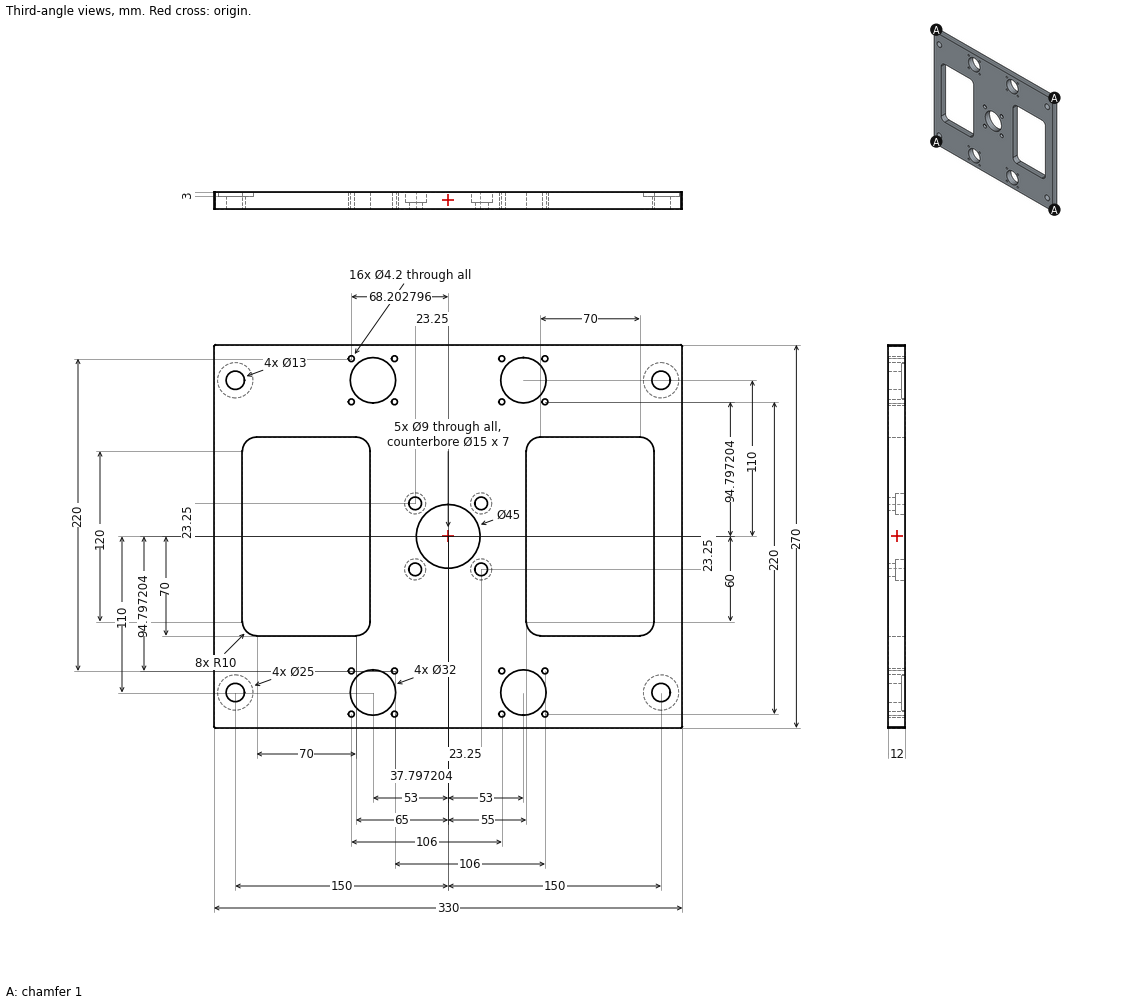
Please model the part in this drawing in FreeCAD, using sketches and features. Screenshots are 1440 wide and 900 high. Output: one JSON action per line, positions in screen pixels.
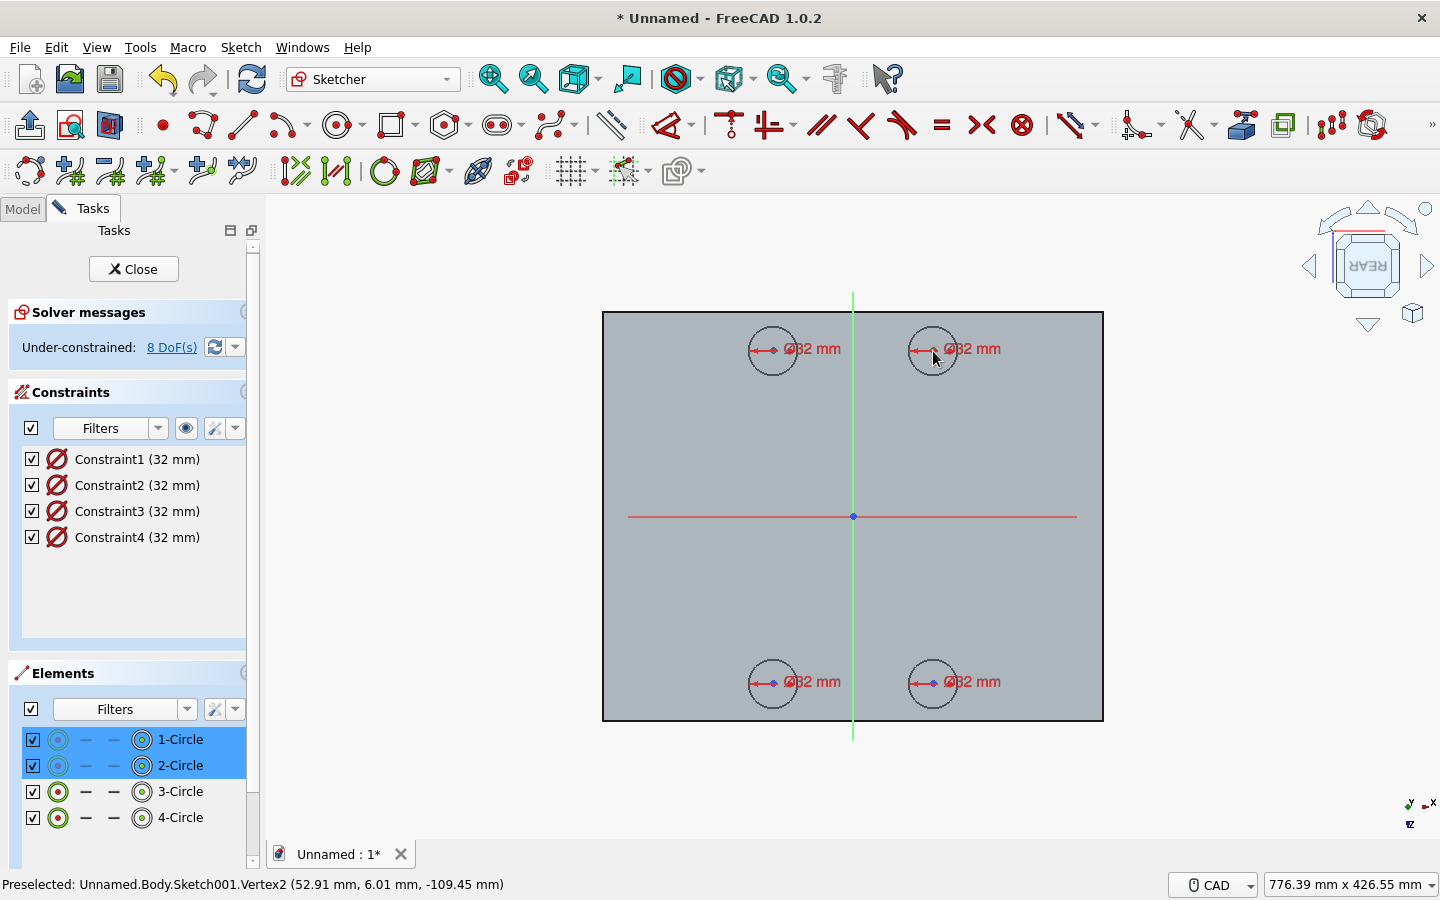
{"action": "left_click", "coordinate": [796, 126]}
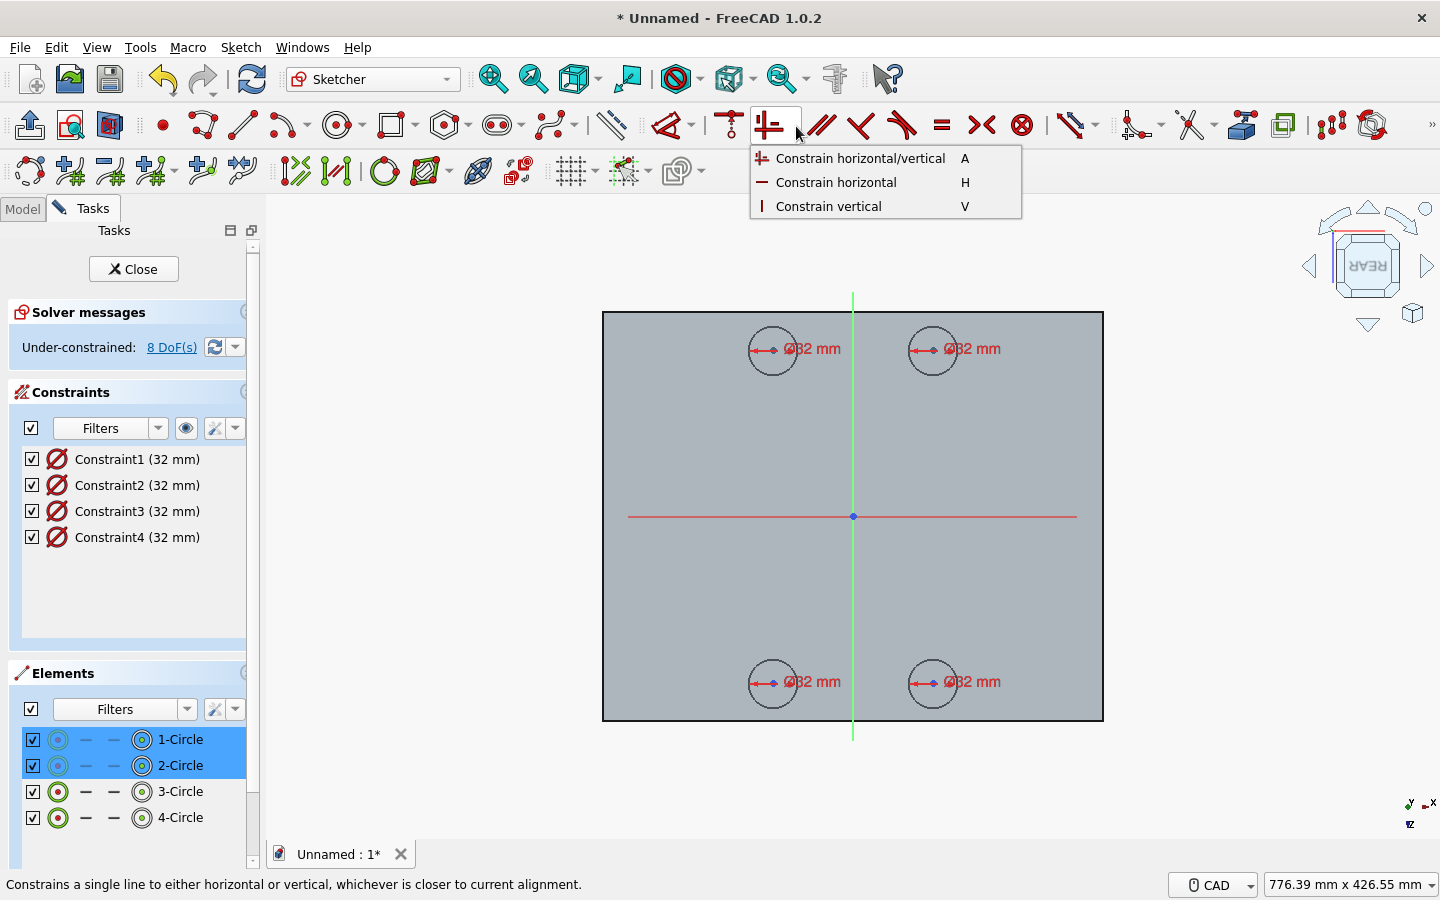
{"action": "left_click", "coordinate": [886, 182]}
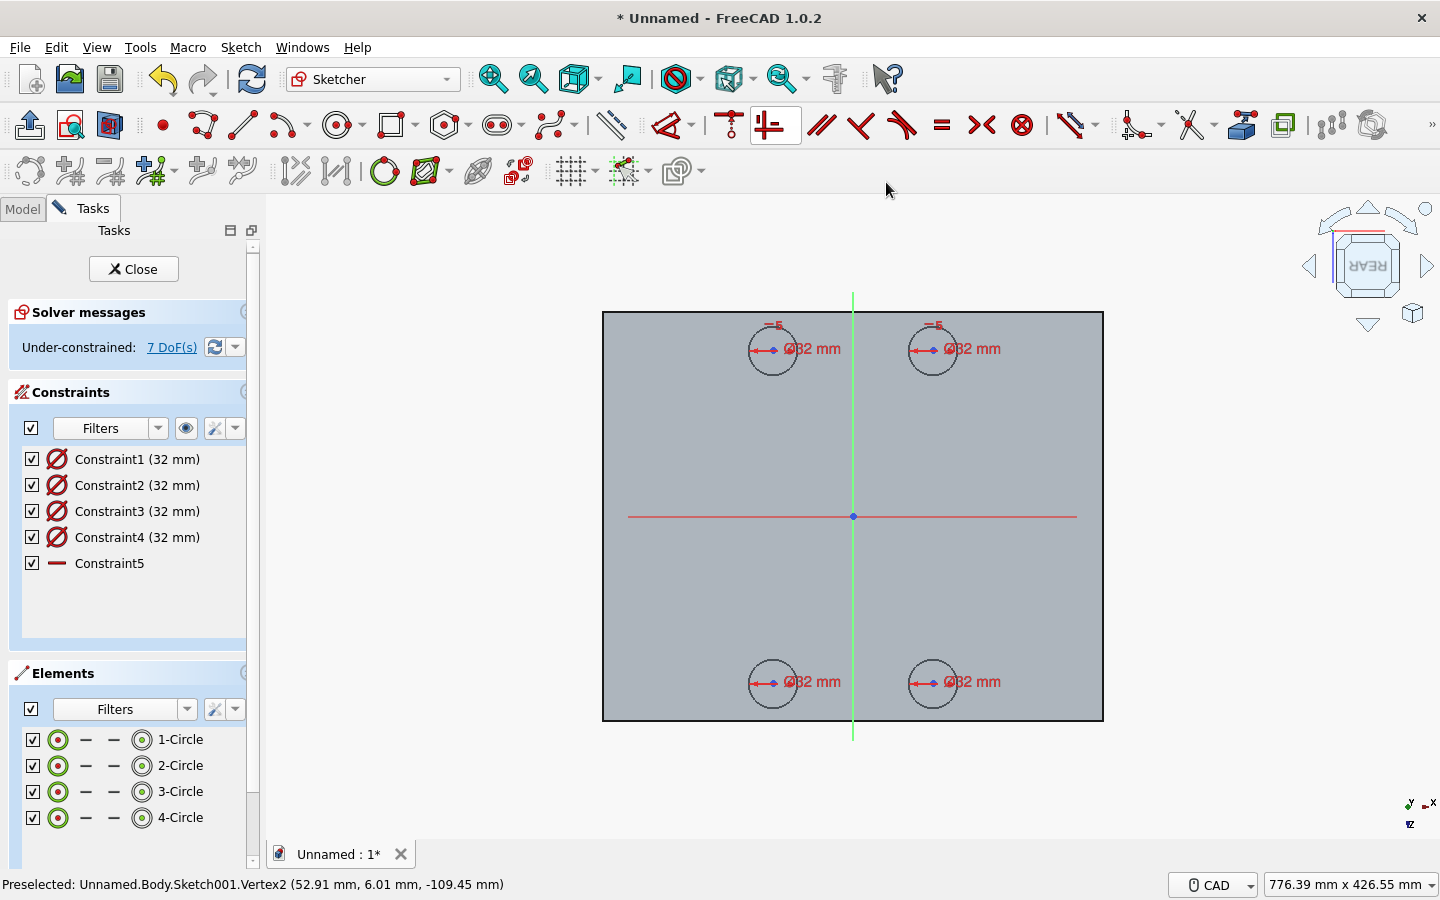
{"action": "left_click", "coordinate": [933, 351]}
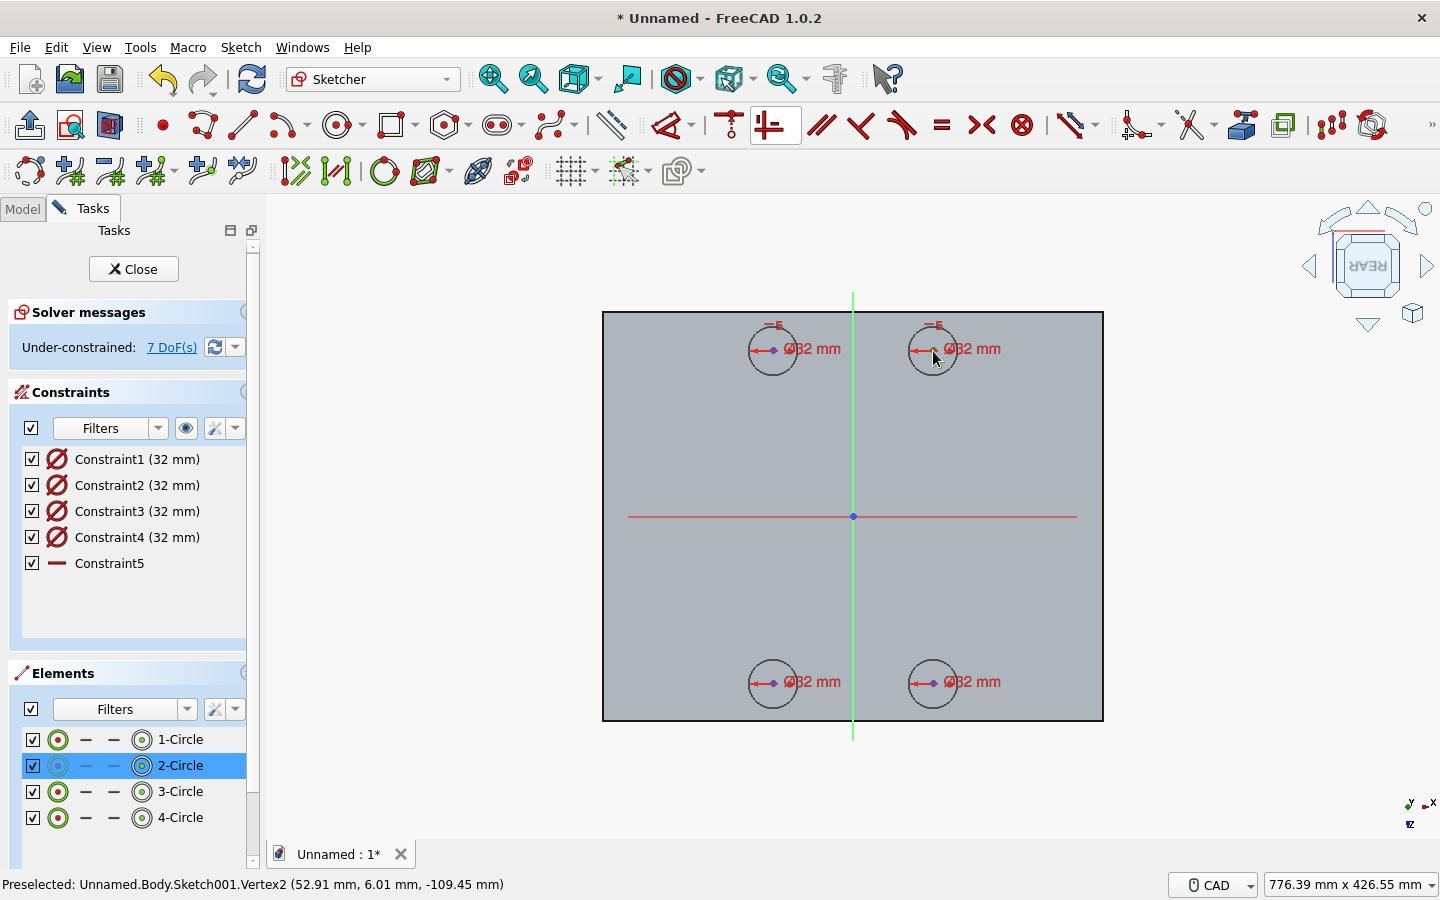
{"action": "left_click", "coordinate": [933, 684]}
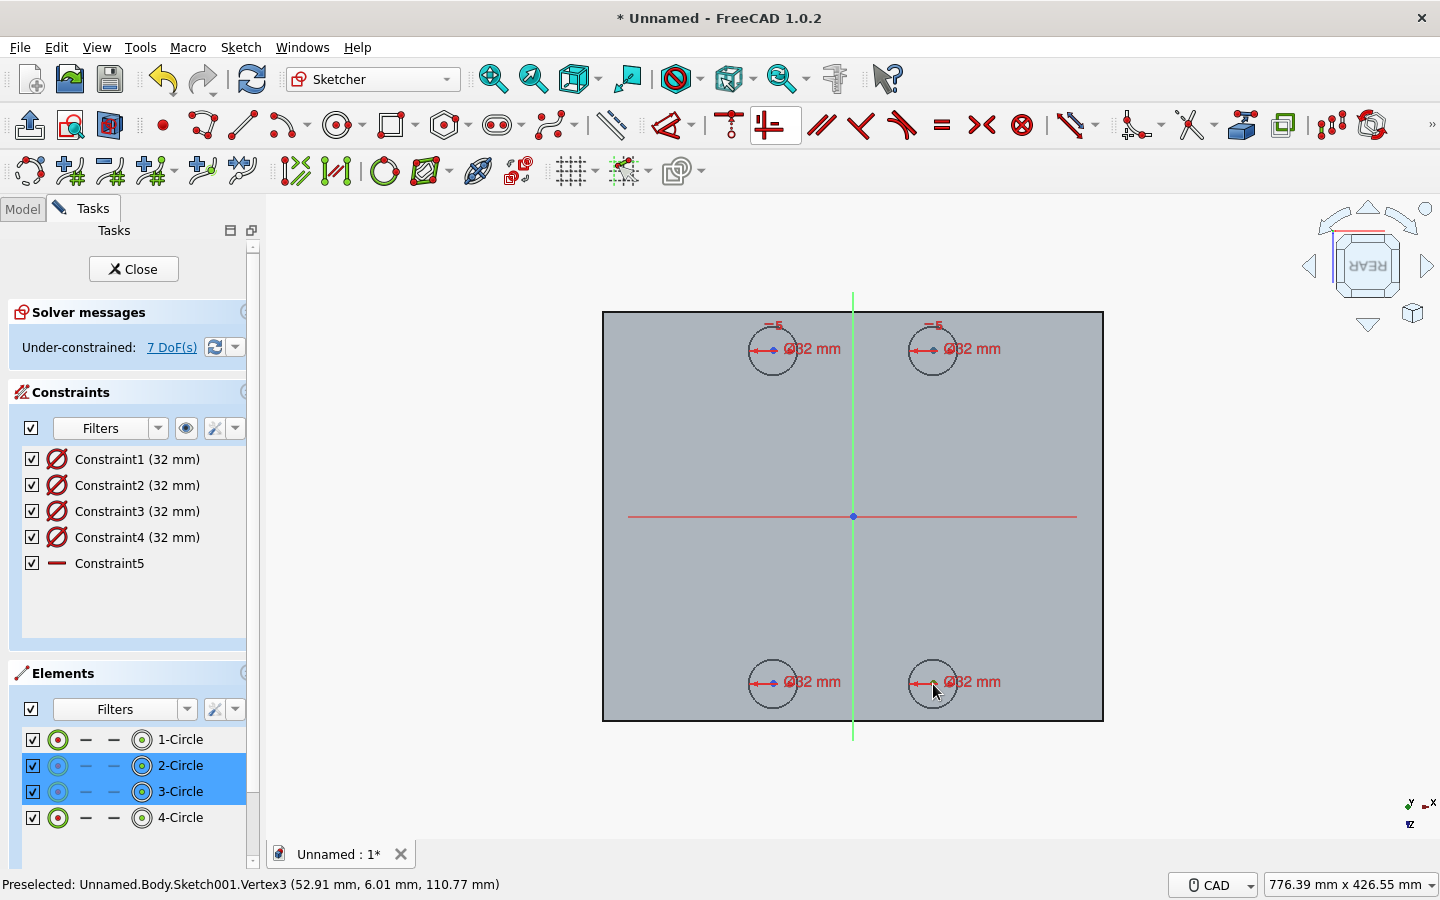
{"action": "key", "text": "v"}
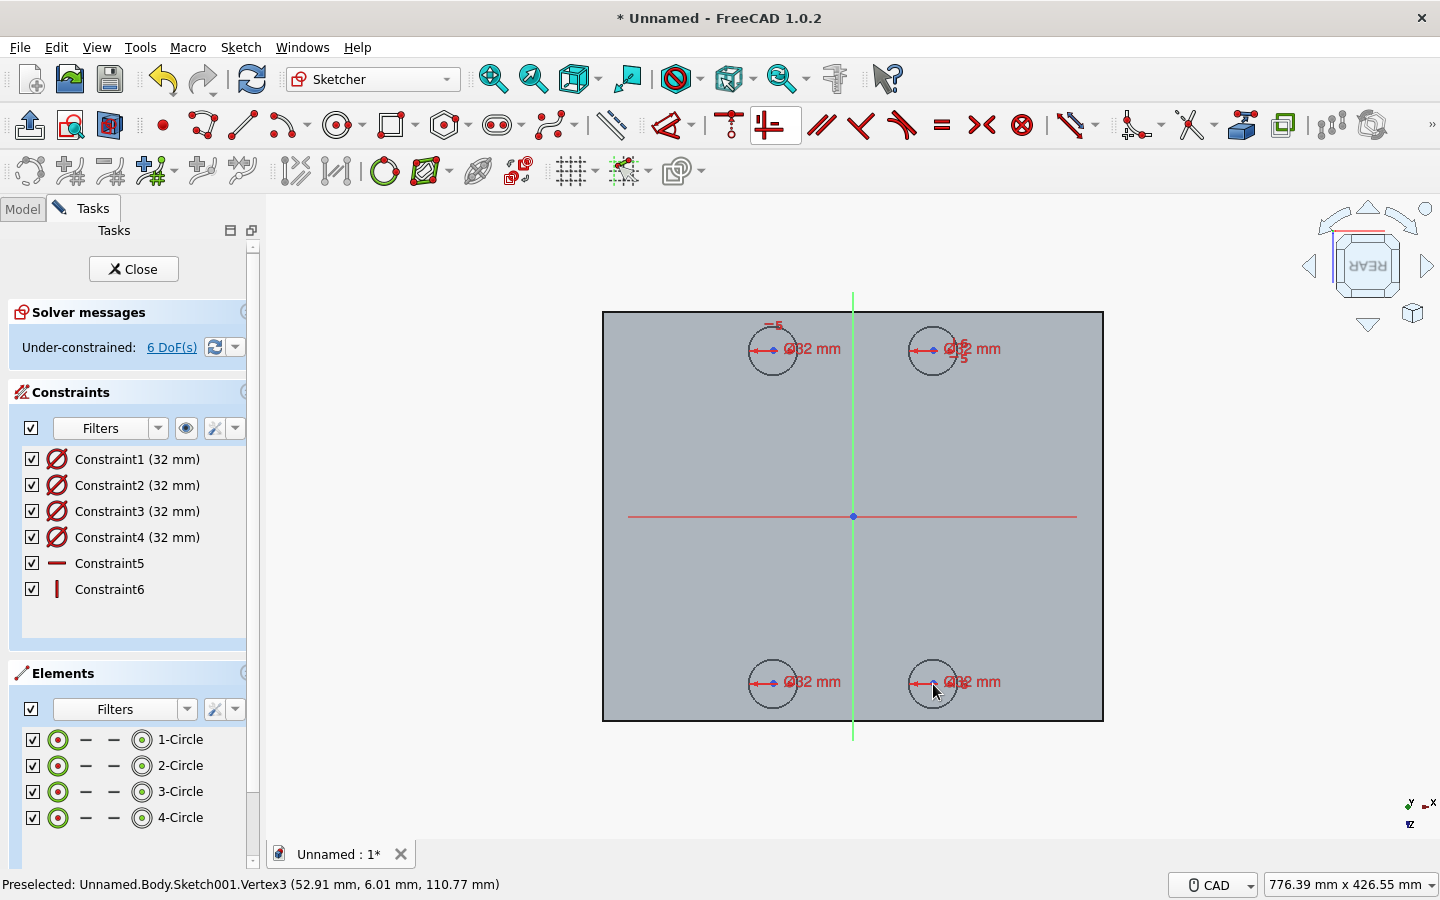
{"action": "left_click", "coordinate": [773, 351]}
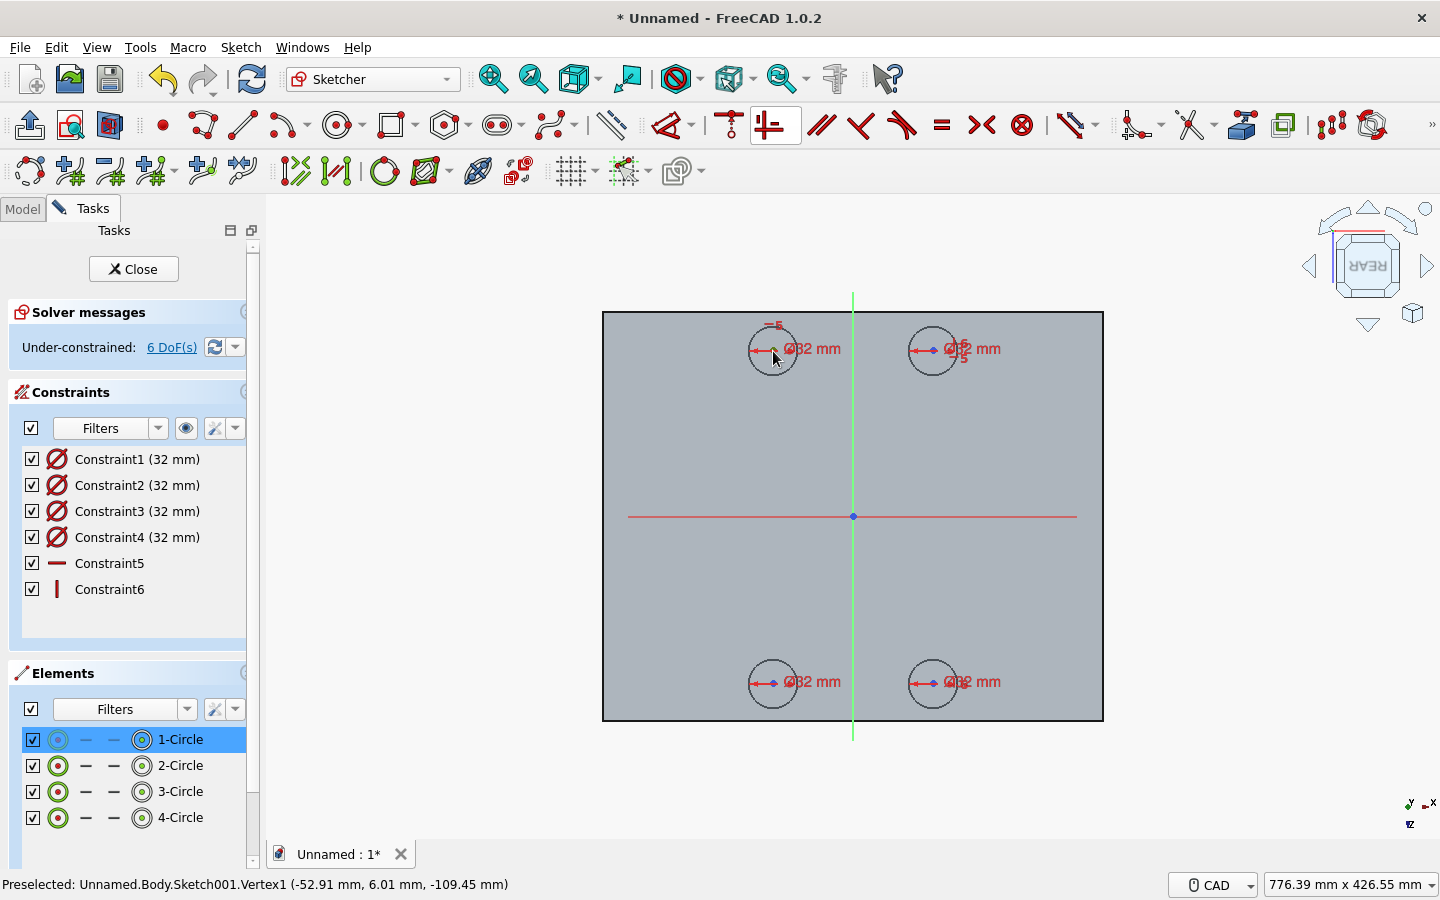
{"action": "left_click", "coordinate": [773, 684]}